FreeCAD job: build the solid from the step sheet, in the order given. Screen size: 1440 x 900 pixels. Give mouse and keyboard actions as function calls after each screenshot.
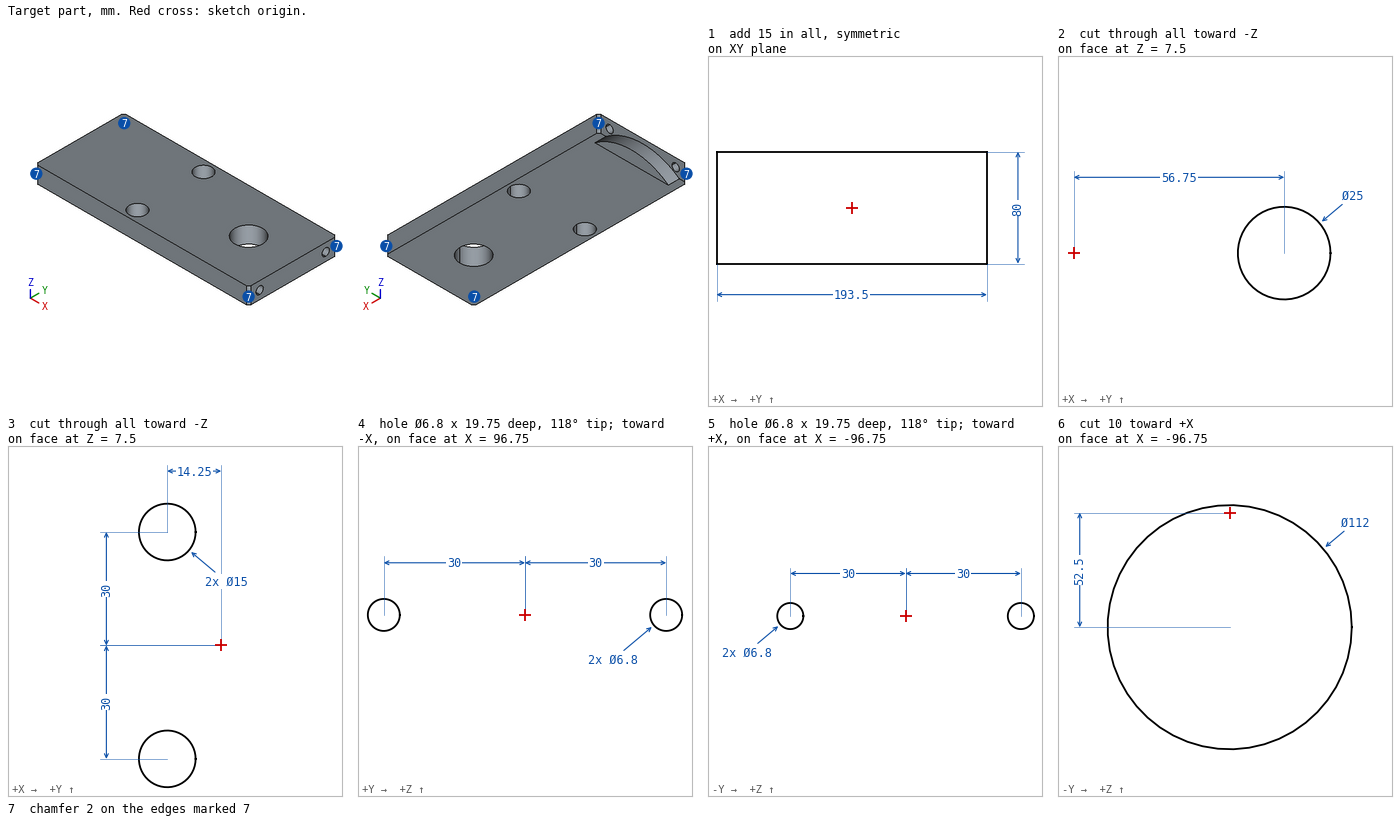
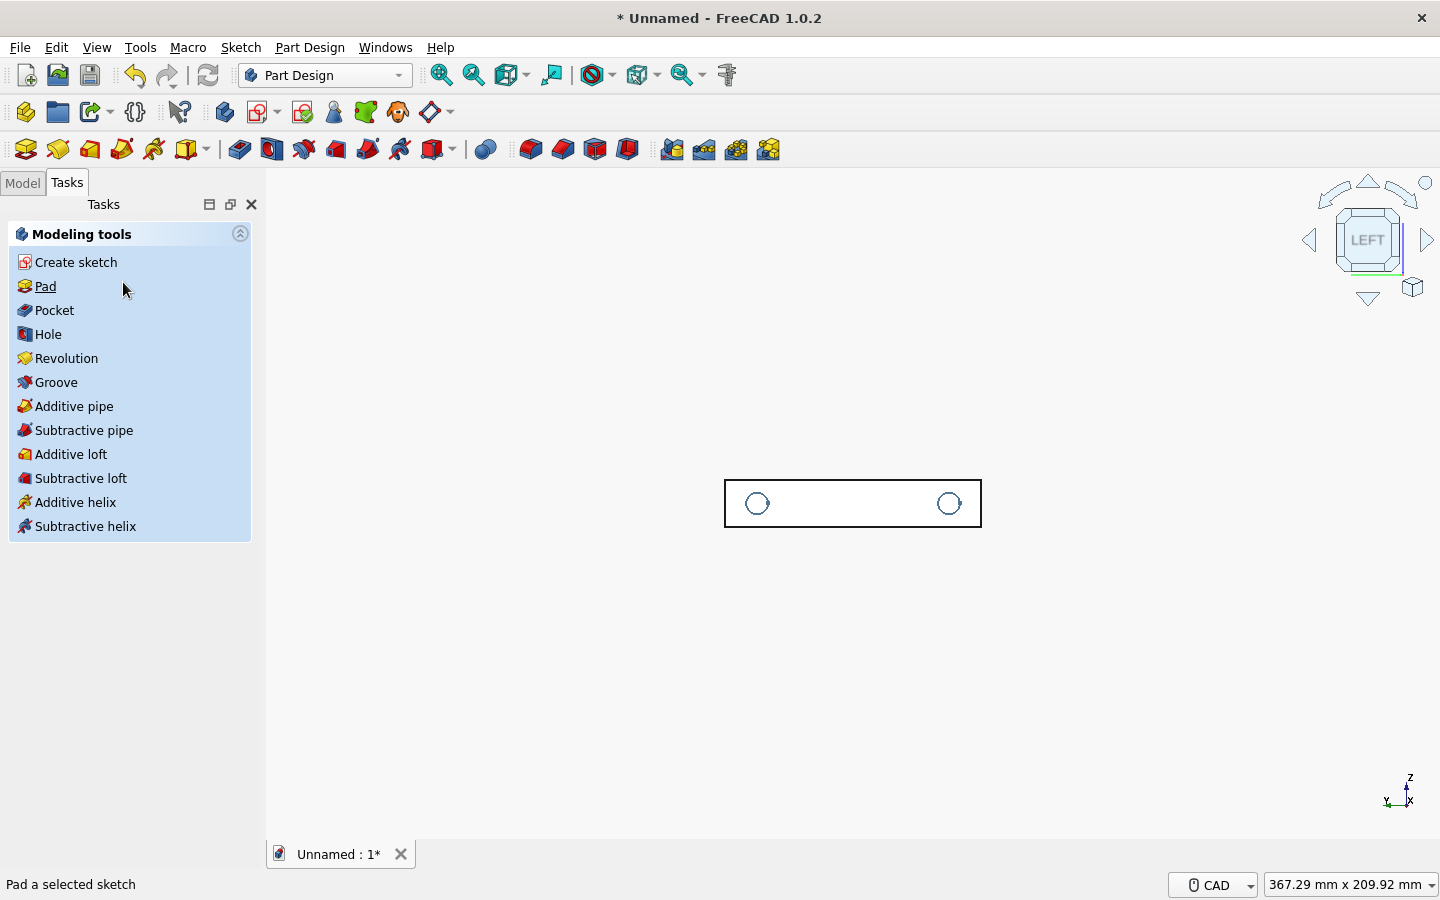
click(272, 150)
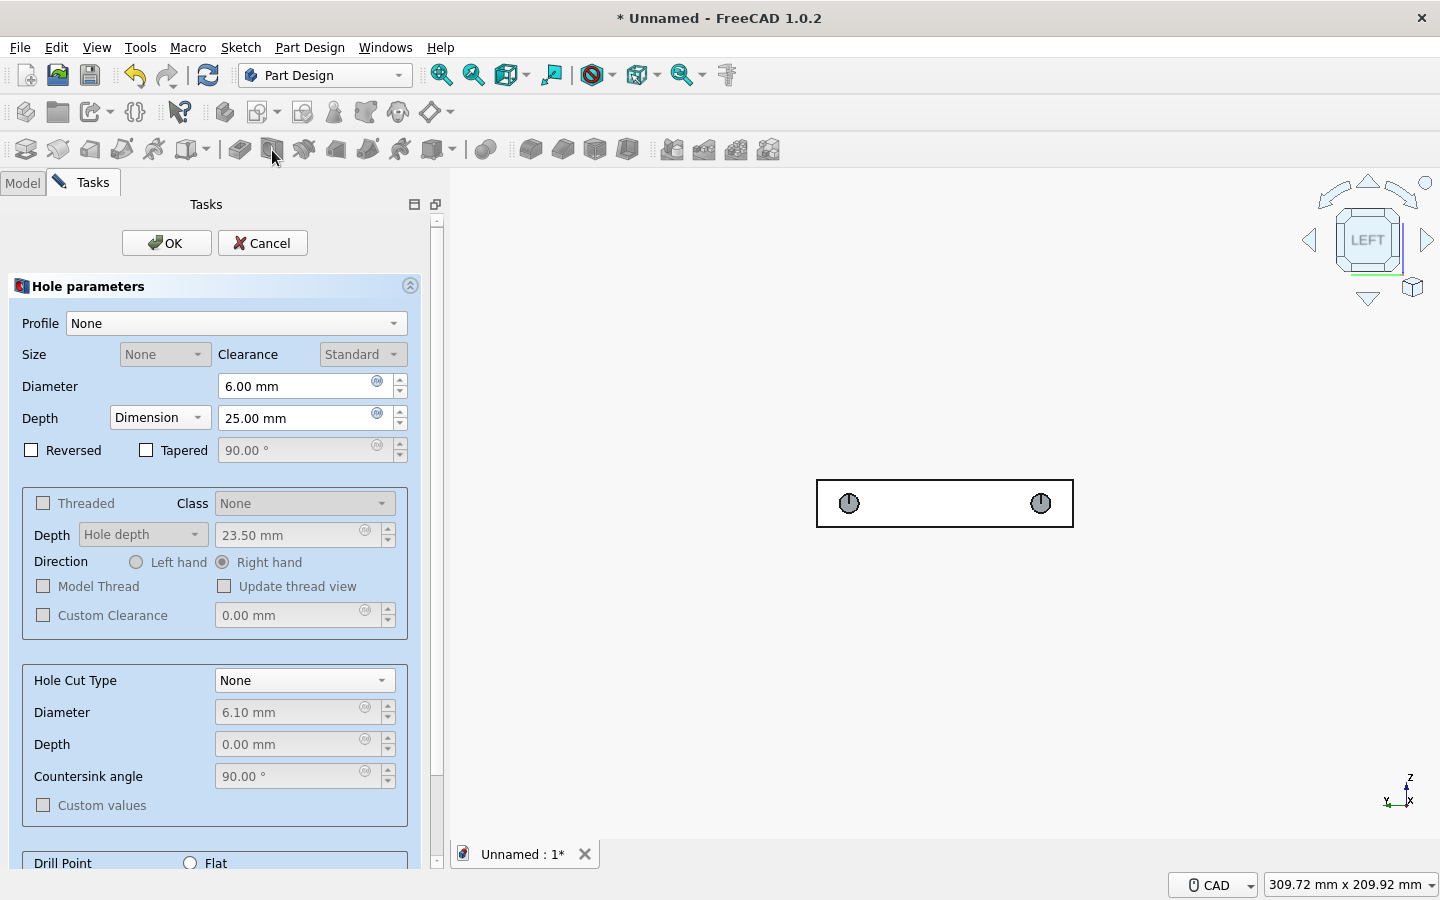
triple_click(305, 386)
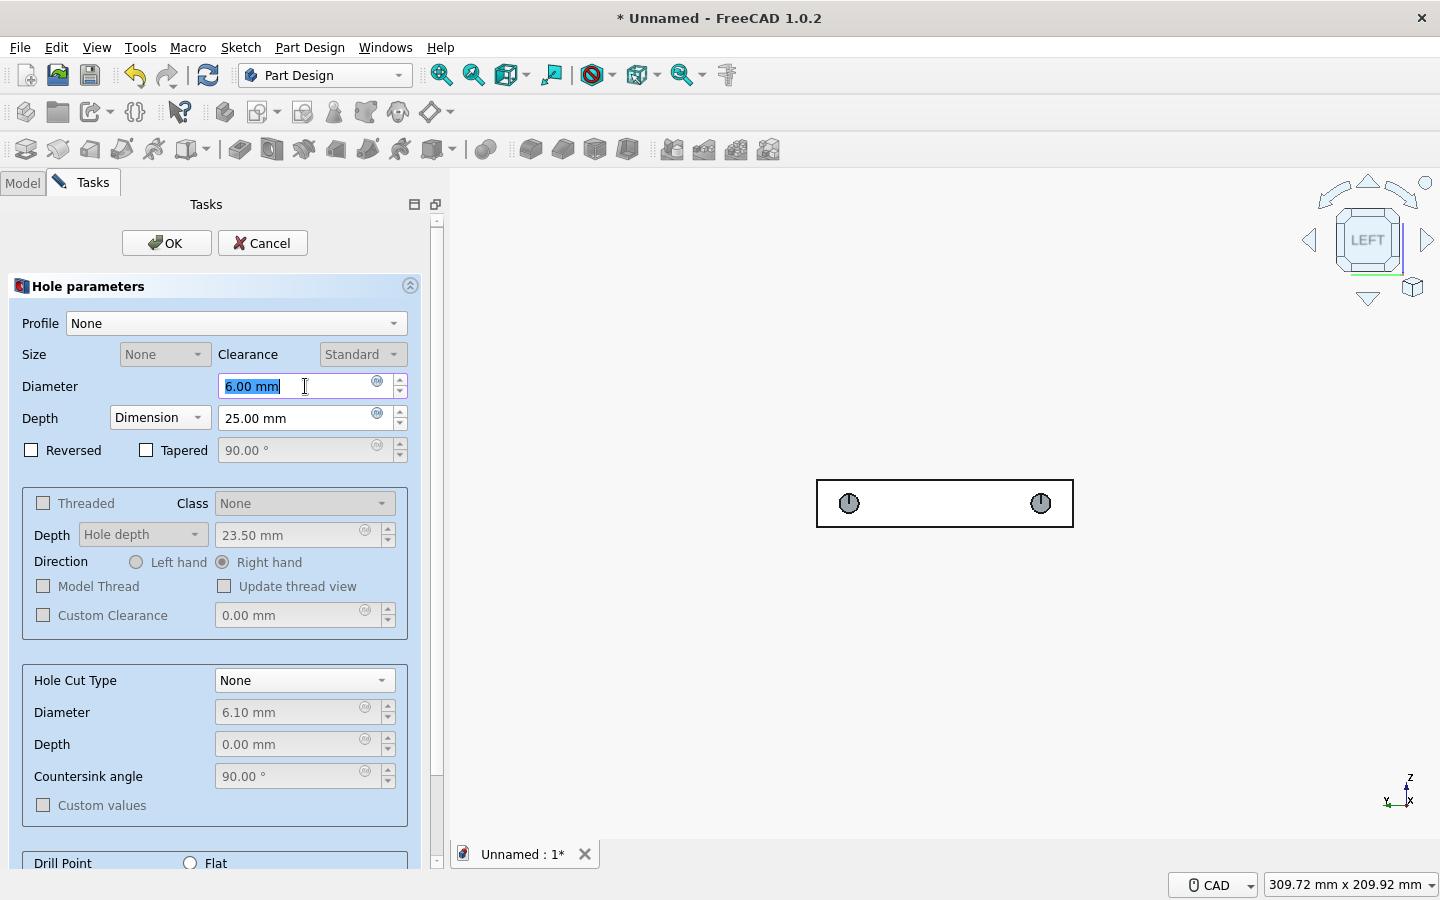
text(6.8)
key(Tab)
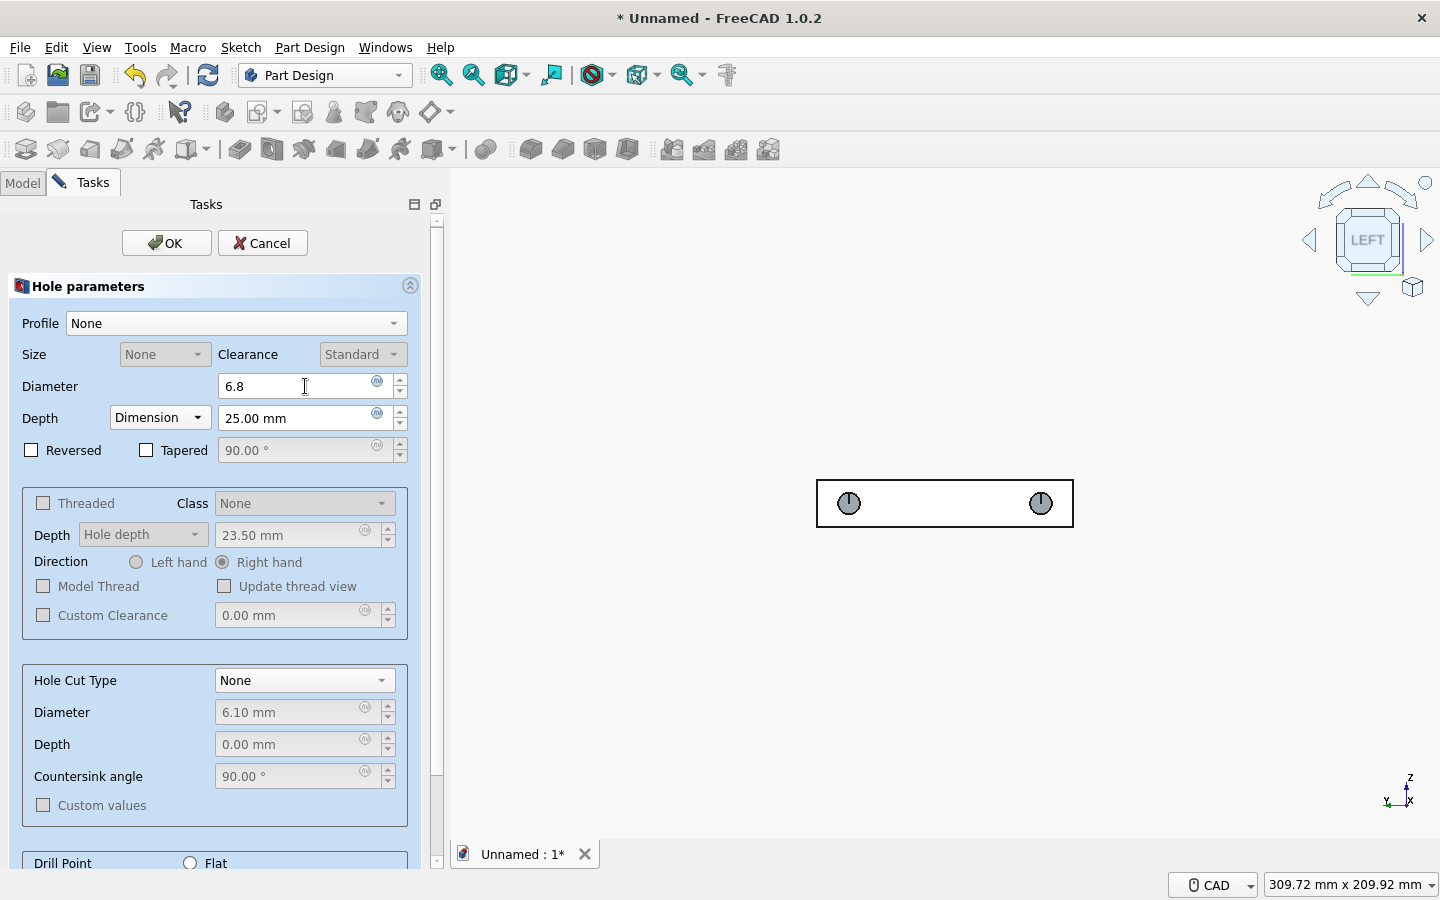
triple_click(305, 418)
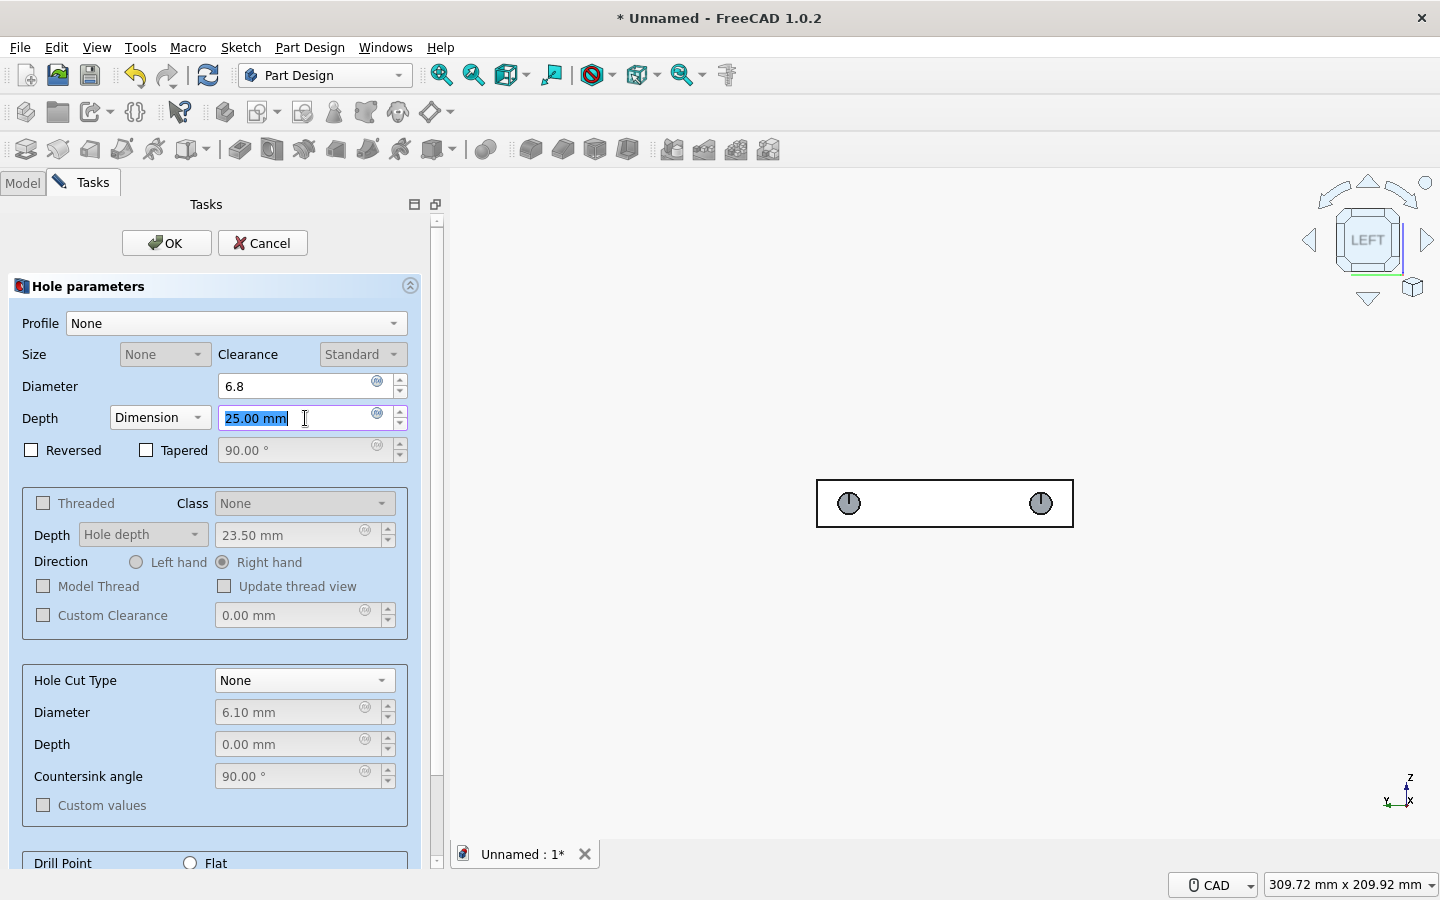
text(19.75)
key(Tab)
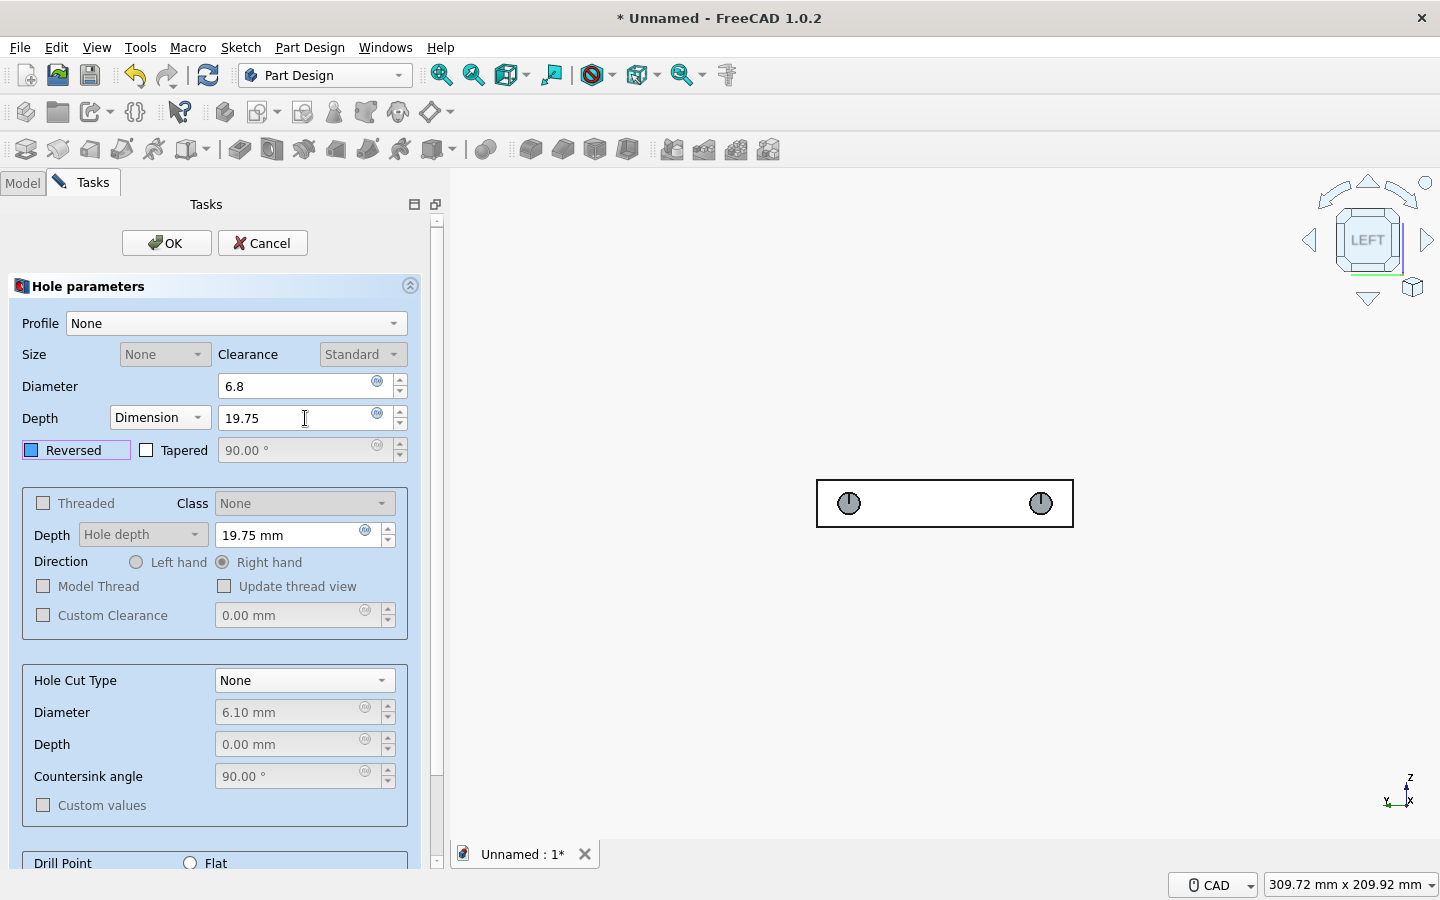
click(167, 243)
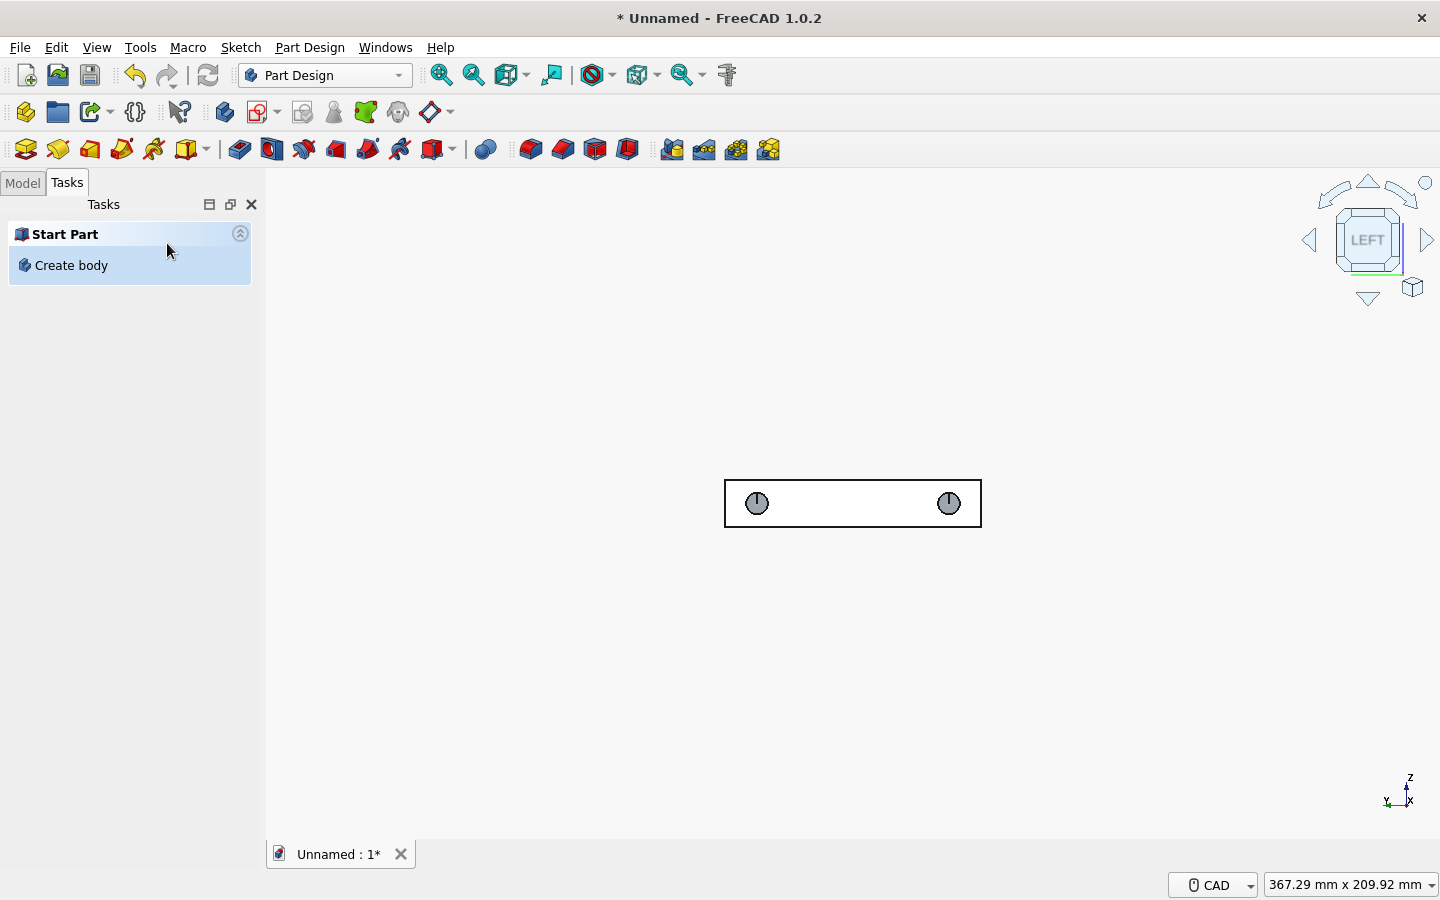
click(442, 76)